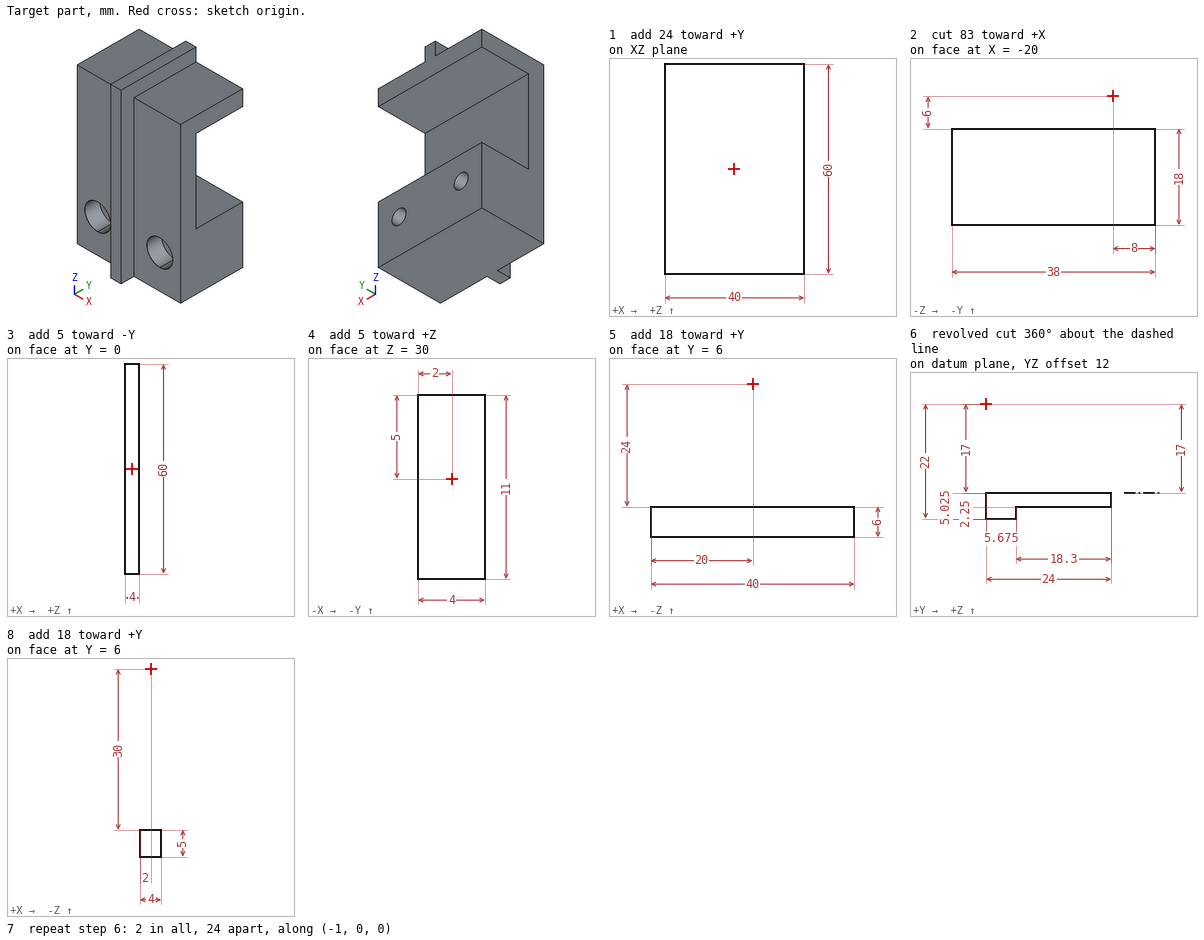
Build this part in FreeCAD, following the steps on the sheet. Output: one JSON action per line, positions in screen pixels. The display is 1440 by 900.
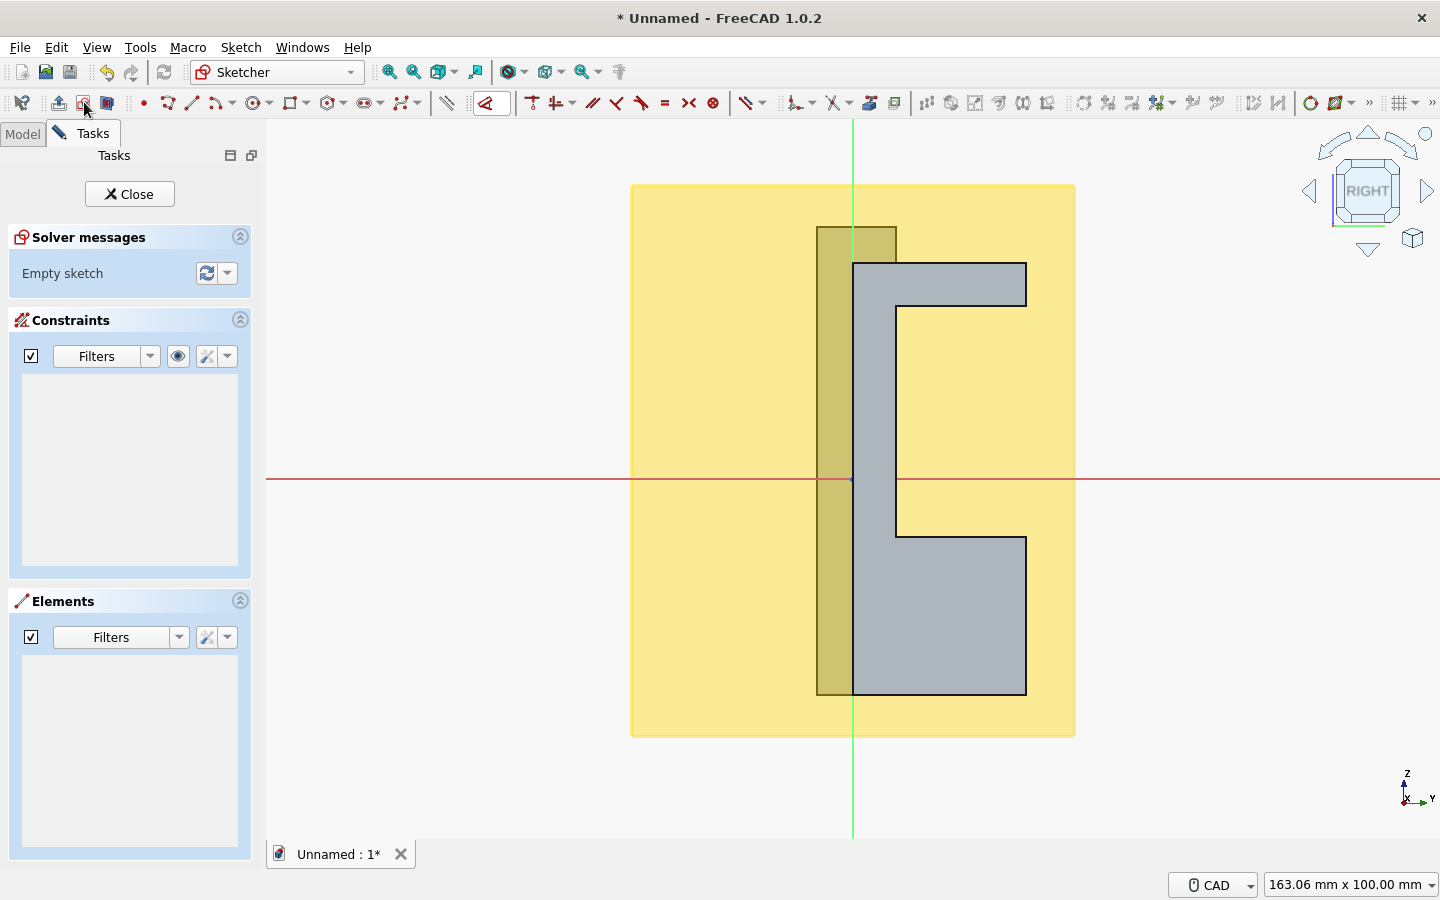
{"action": "left_click", "coordinate": [108, 104]}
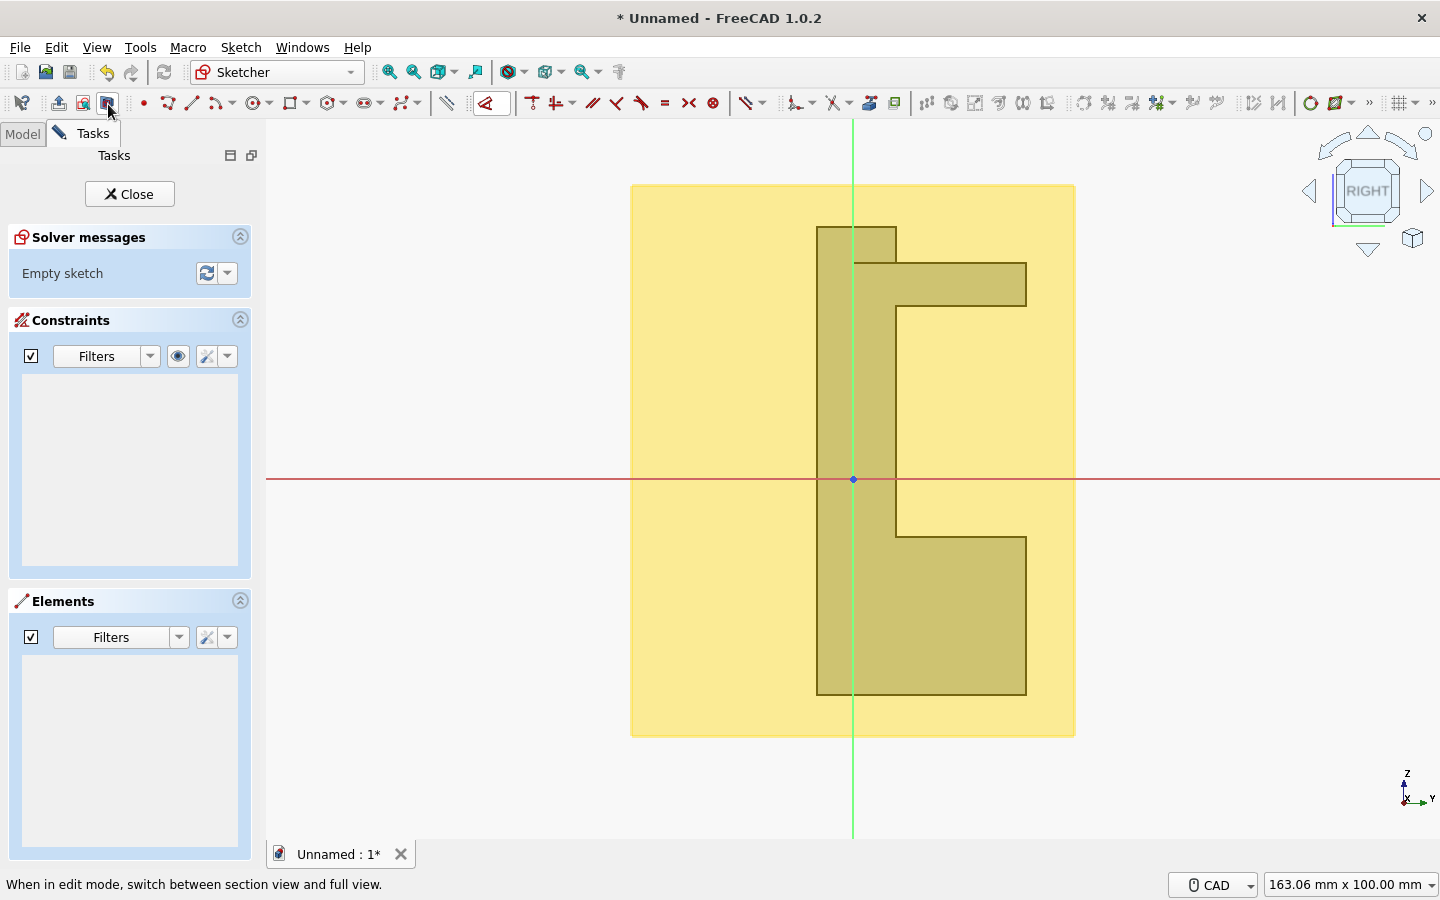
{"action": "scroll", "coordinate": [1084, 604], "scroll_direction": "up", "scroll_amount": 5}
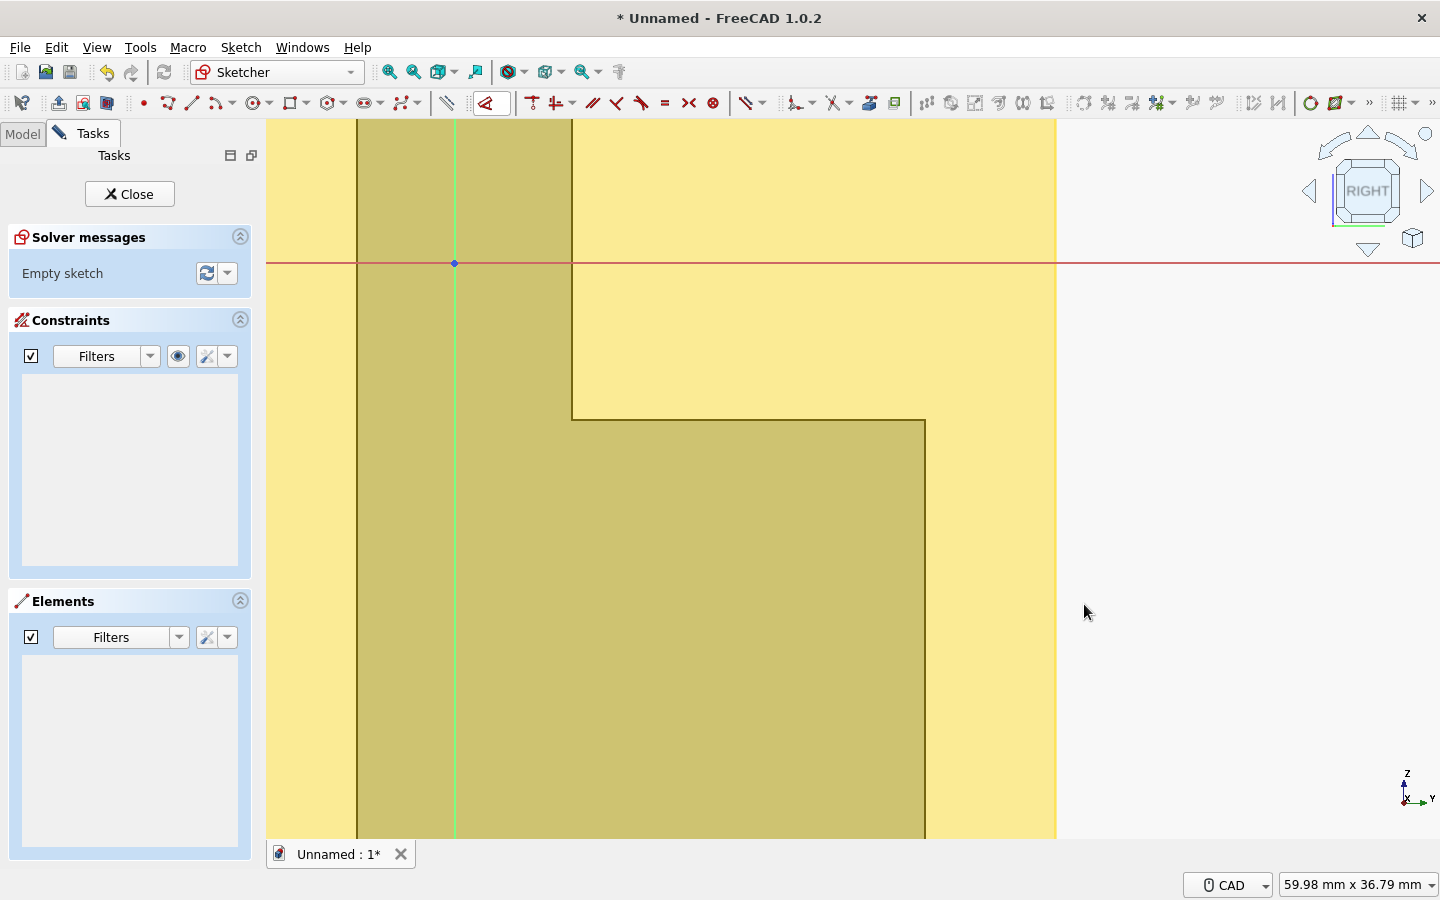
{"action": "key", "text": "g m"}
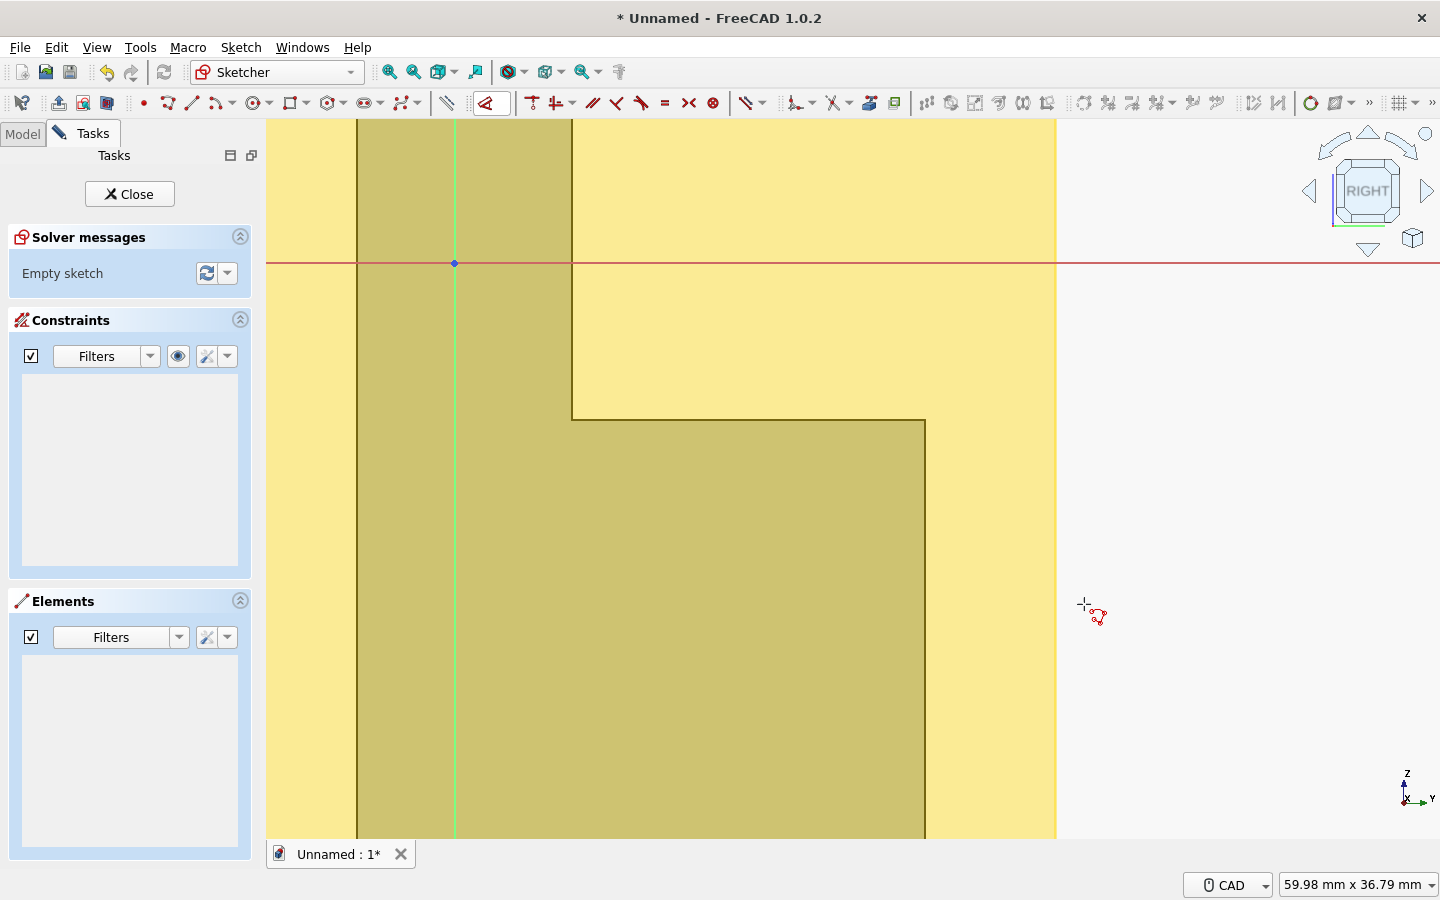
{"action": "left_click", "coordinate": [455, 596]}
{"action": "left_click", "coordinate": [464, 694]}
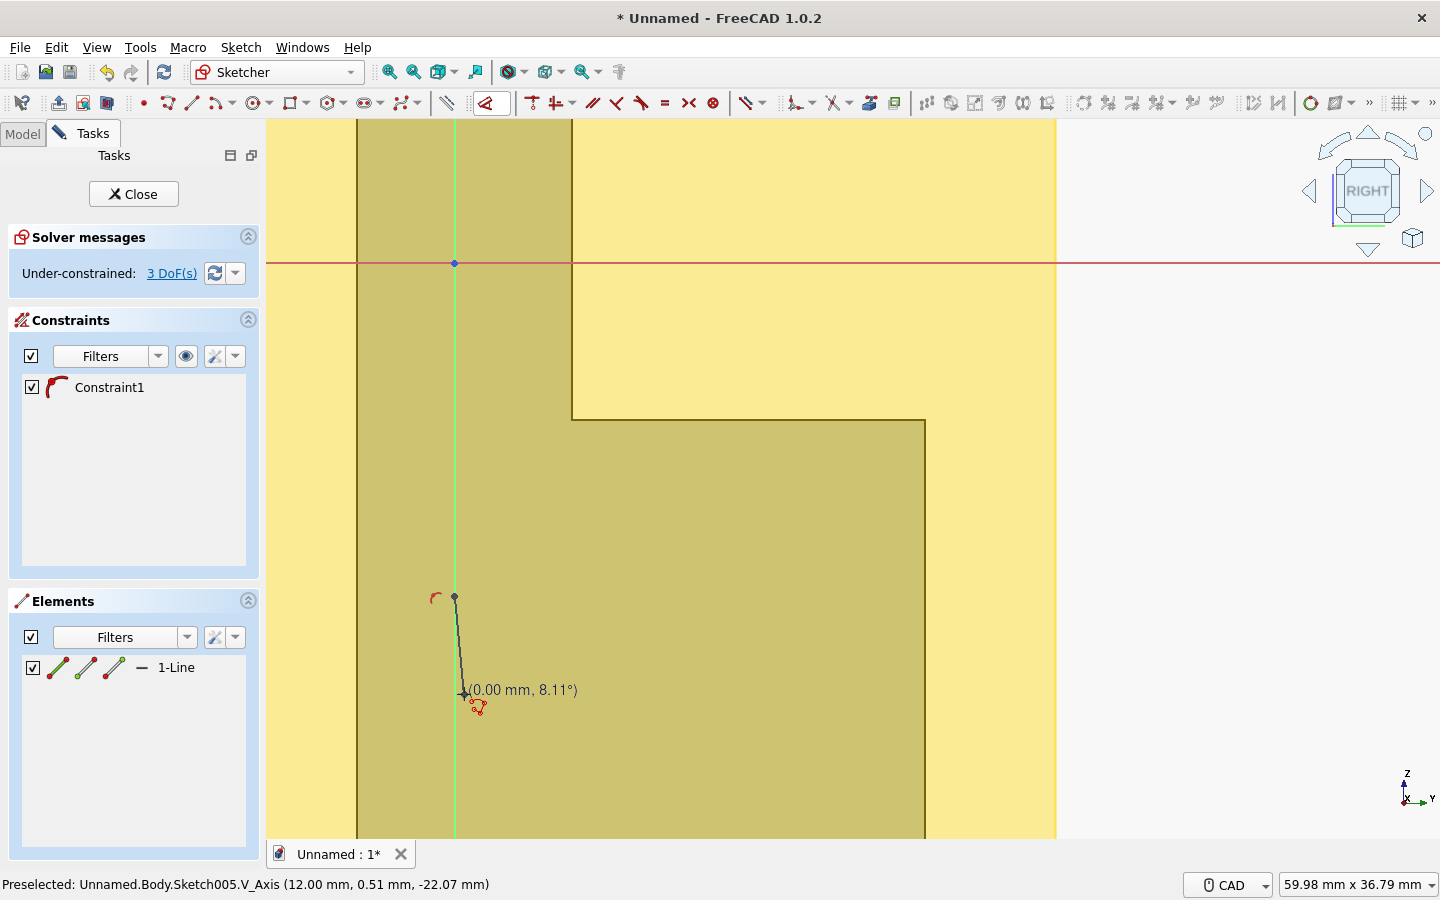
{"action": "scroll", "coordinate": [455, 694], "scroll_direction": "up", "scroll_amount": 18}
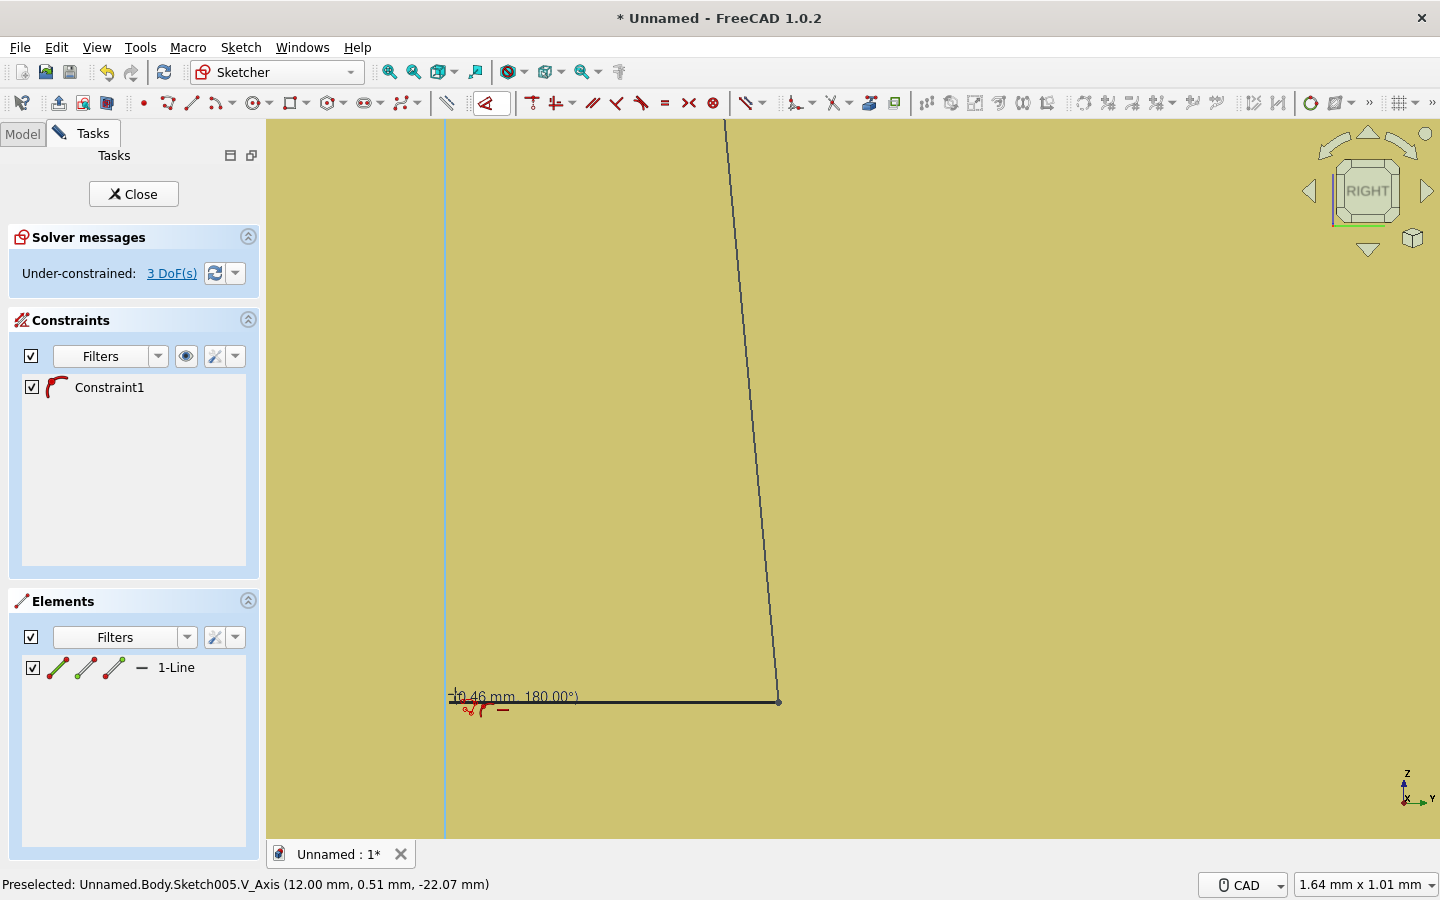
{"action": "left_click", "coordinate": [463, 652]}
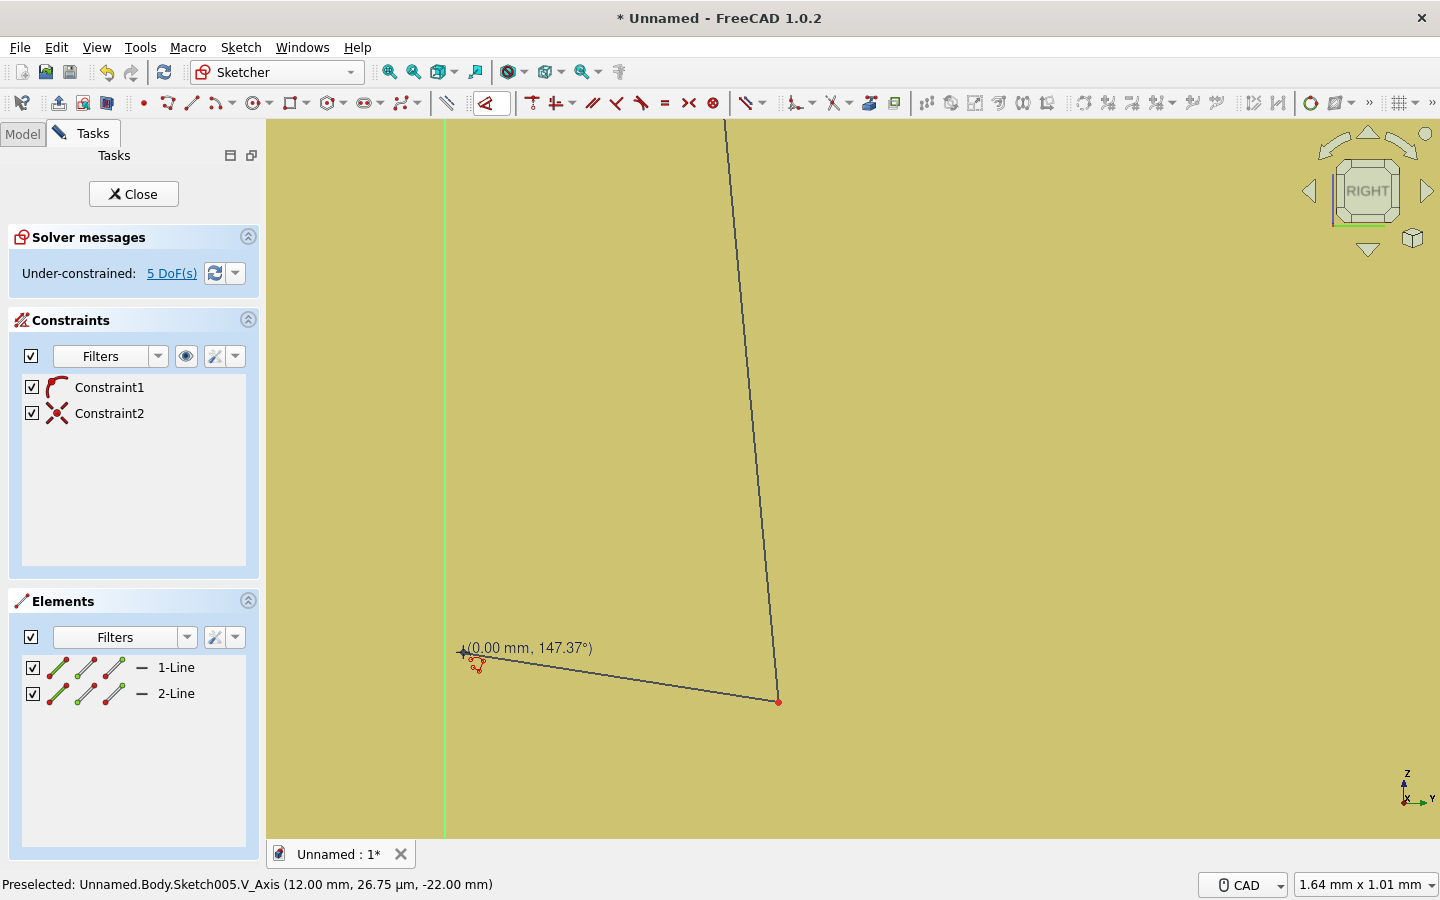
{"action": "scroll", "coordinate": [381, 745], "scroll_direction": "down", "scroll_amount": 17}